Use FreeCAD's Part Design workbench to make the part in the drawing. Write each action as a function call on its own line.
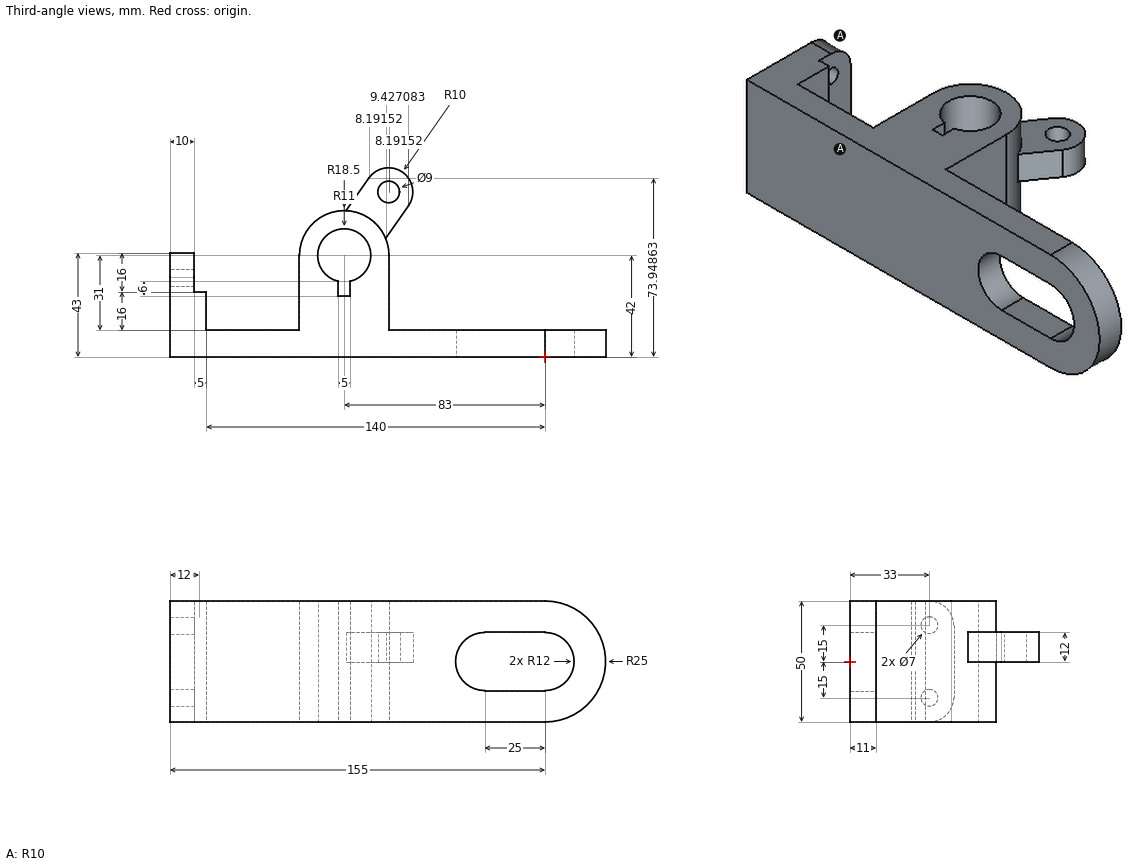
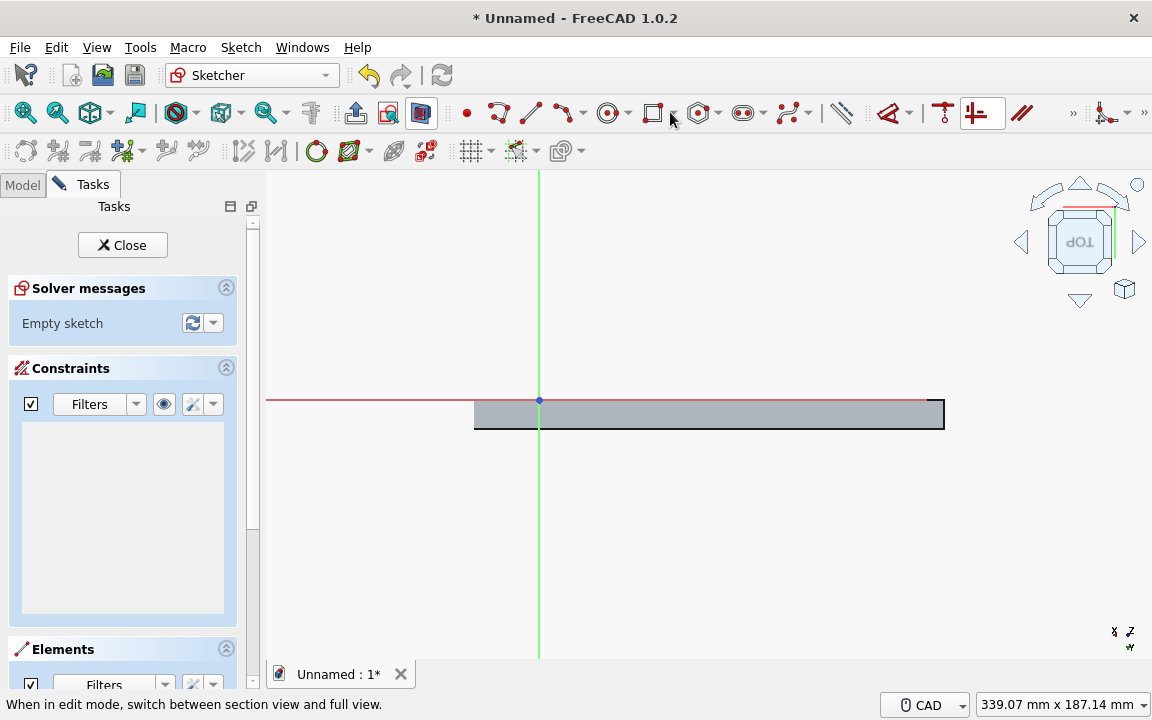
click(500, 114)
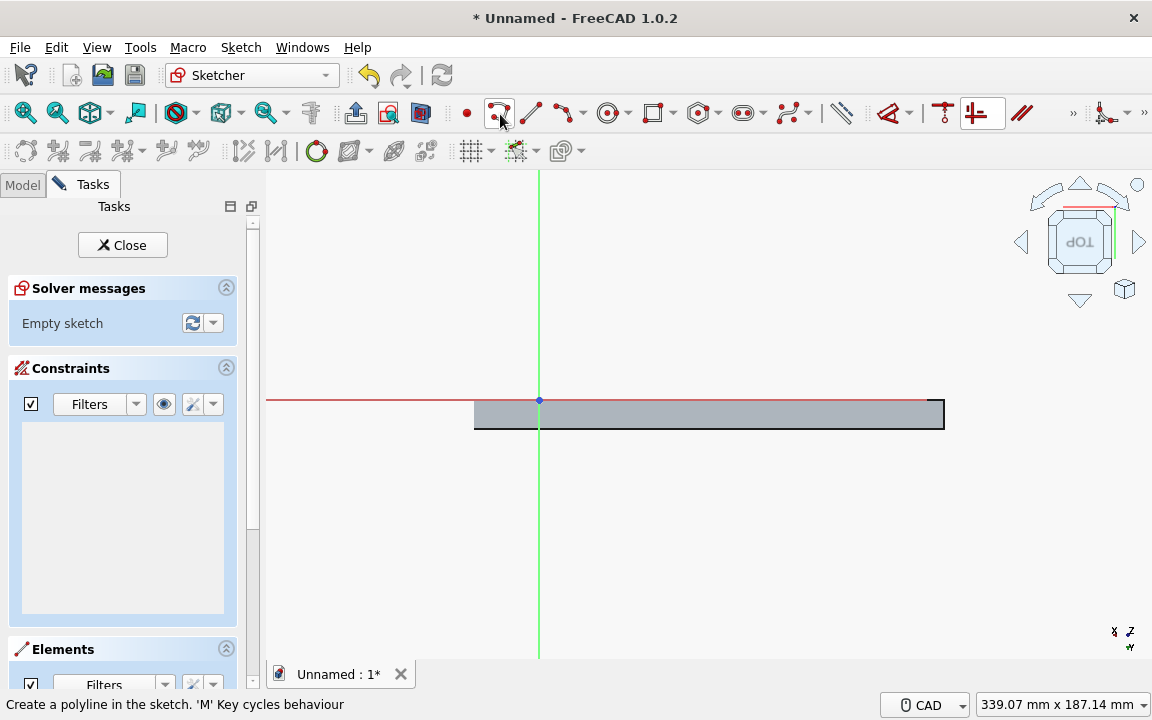
click(905, 429)
click(905, 471)
click(918, 471)
click(918, 512)
click(944, 512)
click(944, 400)
click(905, 430)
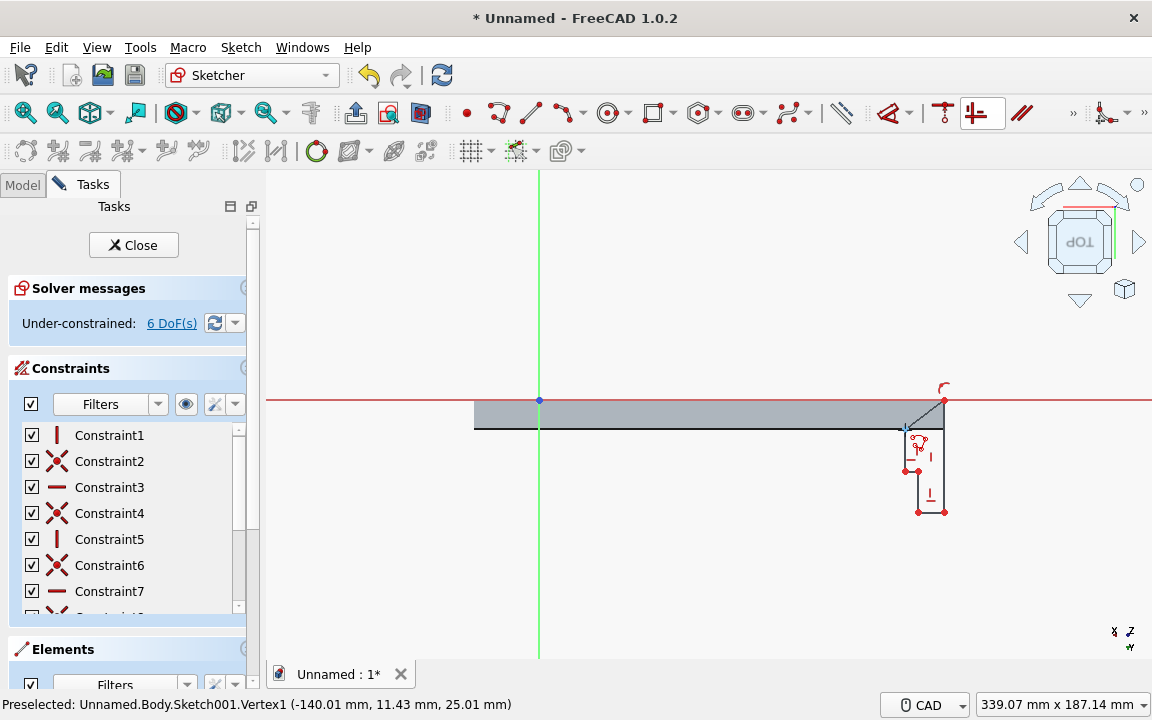
click(804, 510)
click(804, 429)
click(708, 429)
click(708, 510)
right_click(708, 510)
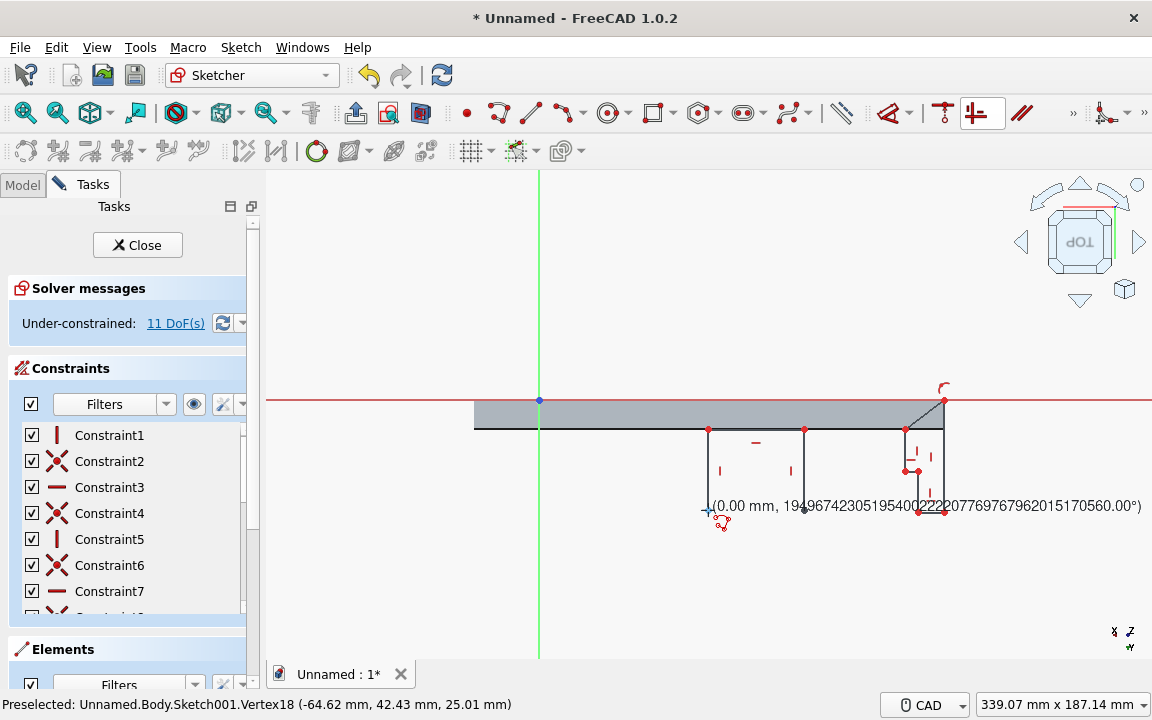
click(564, 114)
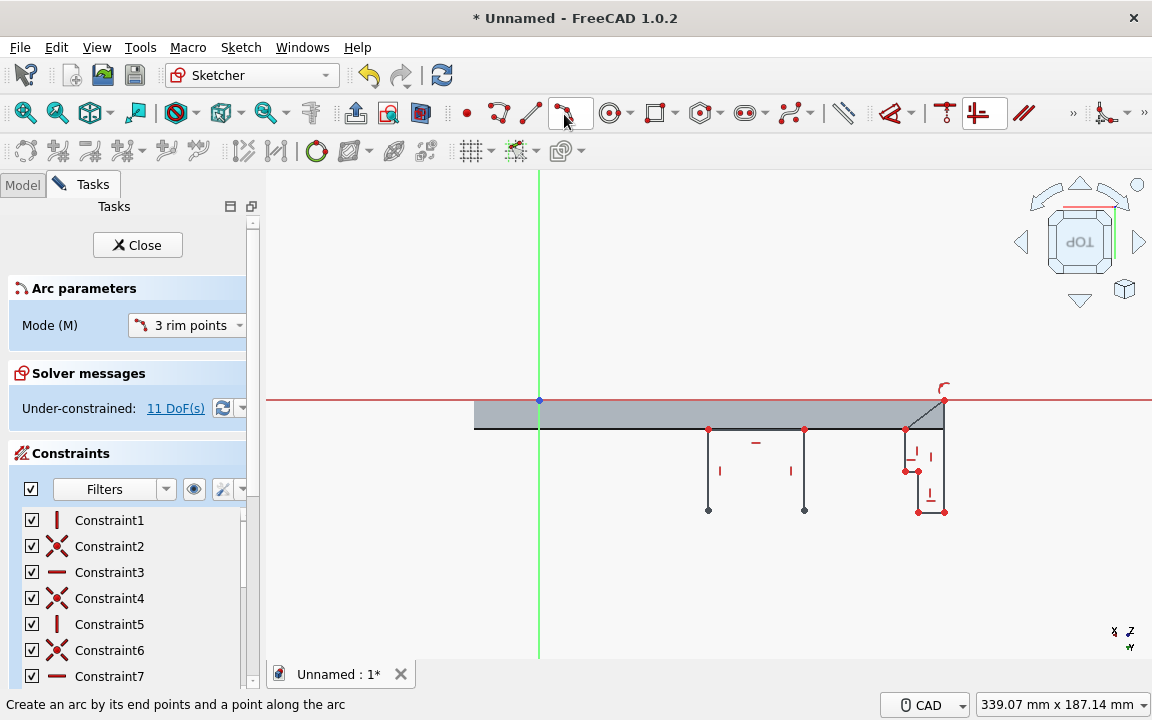
click(708, 511)
click(804, 511)
click(756, 558)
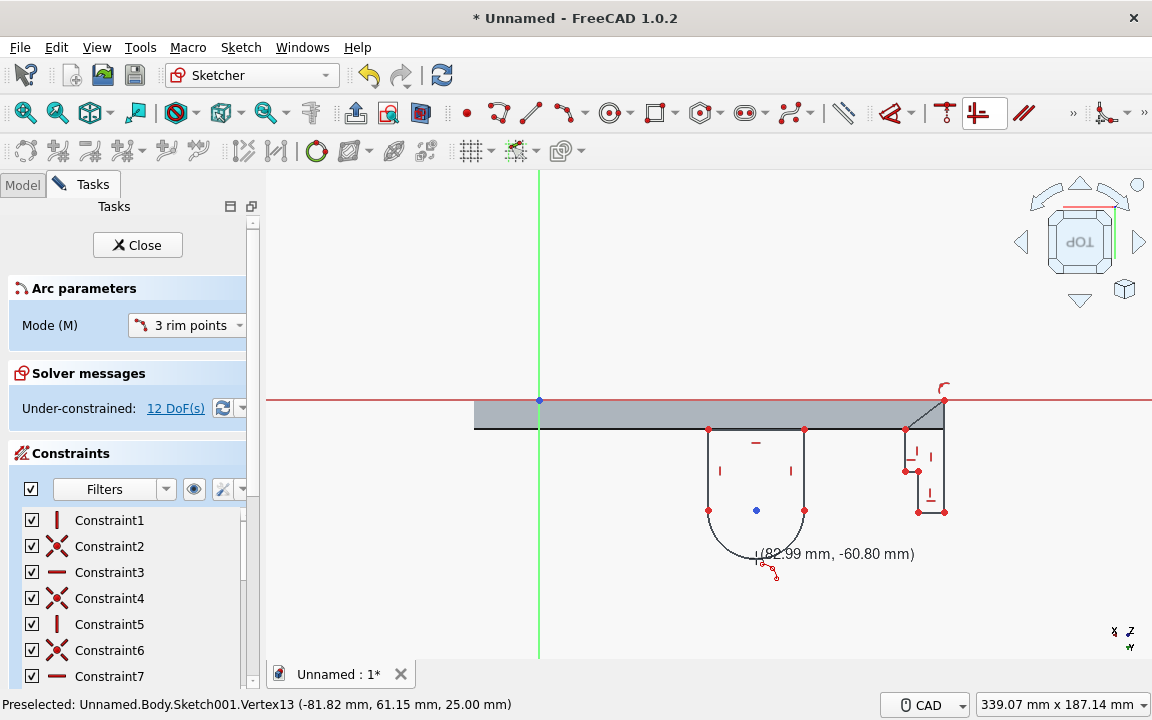
click(500, 114)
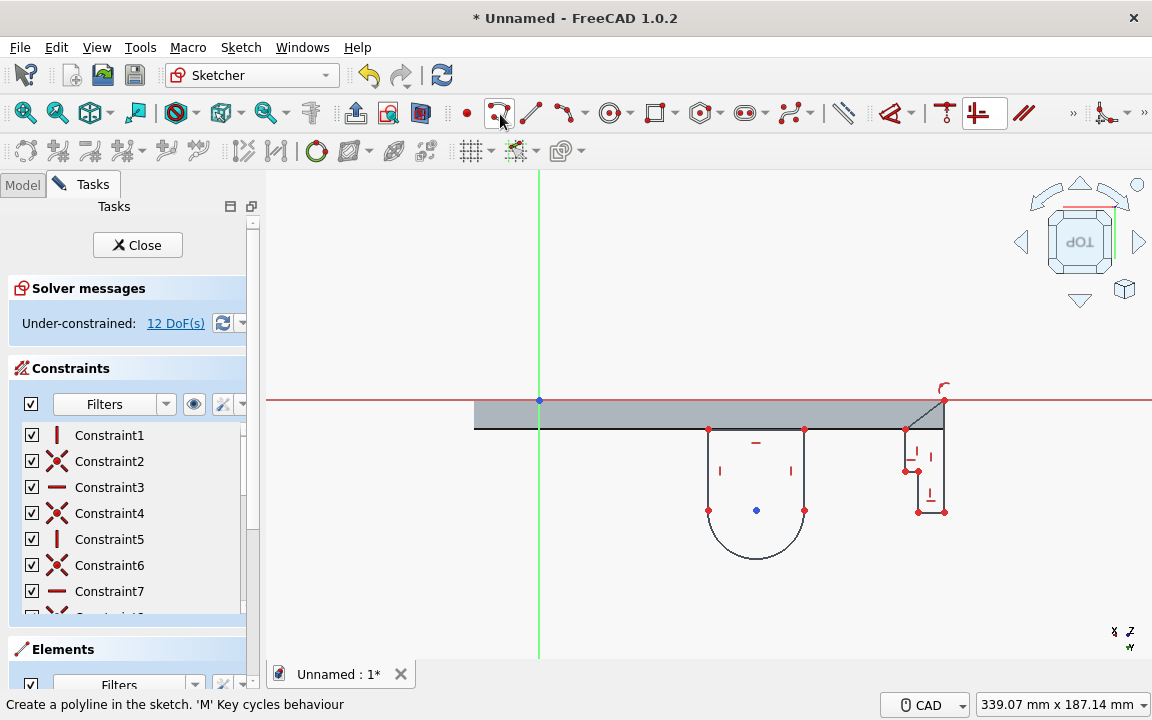
click(750, 482)
click(750, 466)
click(763, 466)
click(763, 482)
right_click(763, 482)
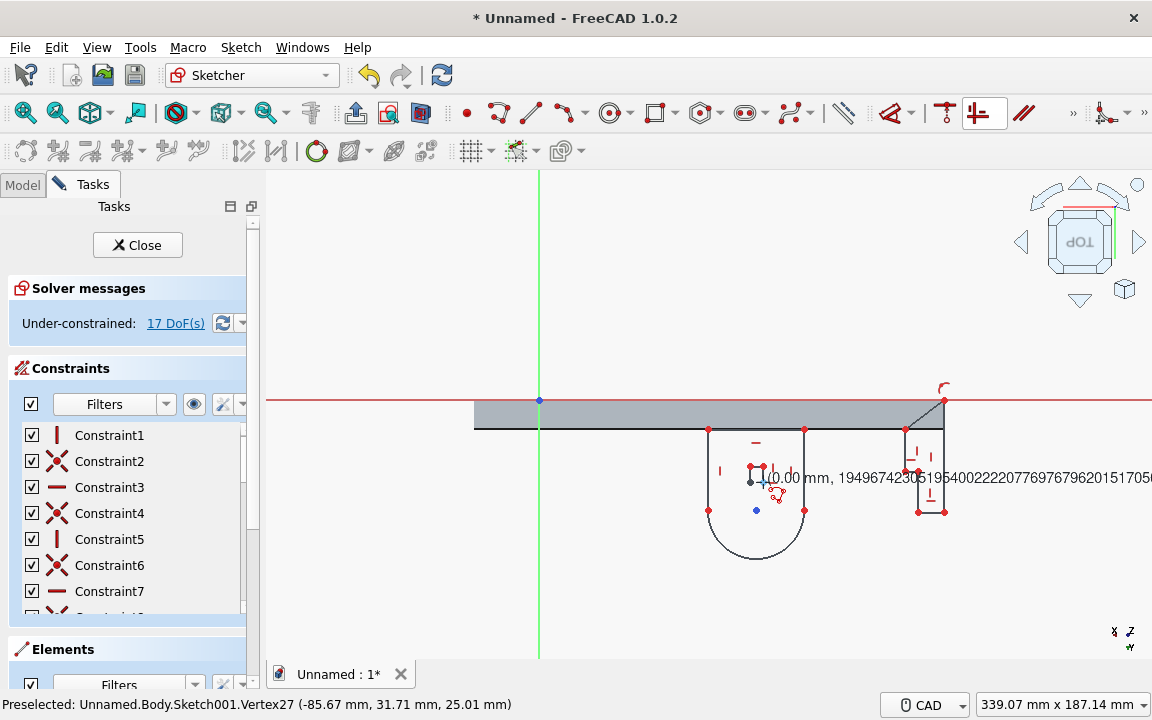
key(g)
key(3)
key(a)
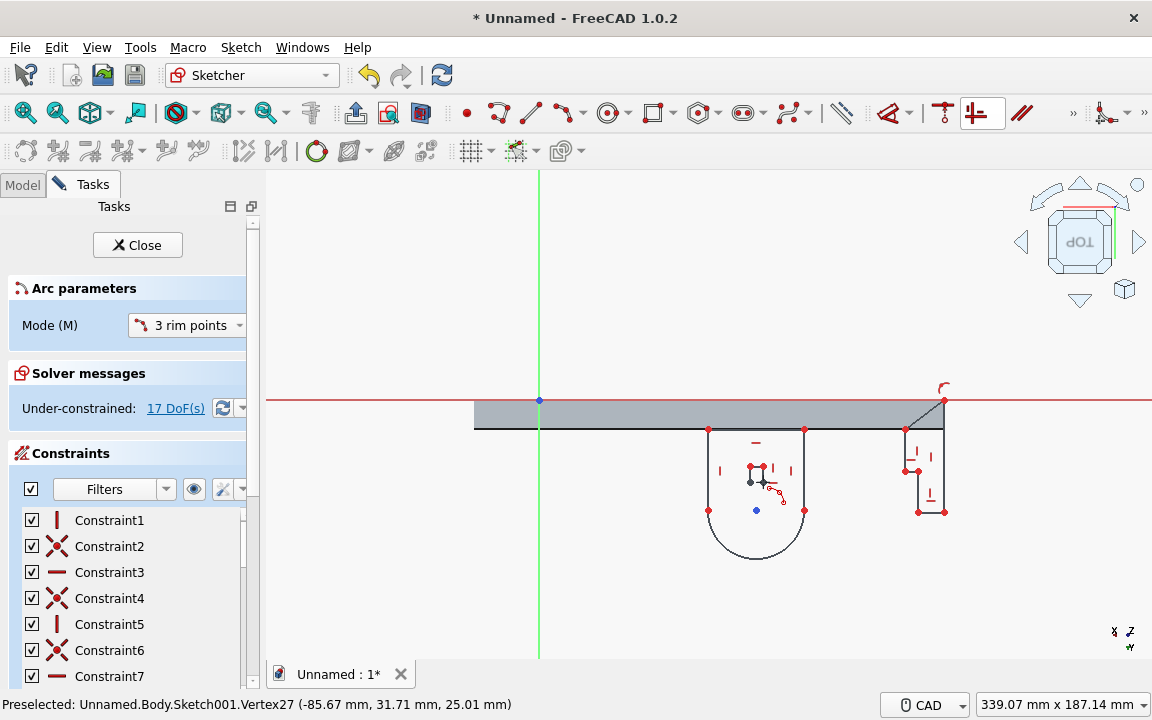
scroll(763, 482, up, 4)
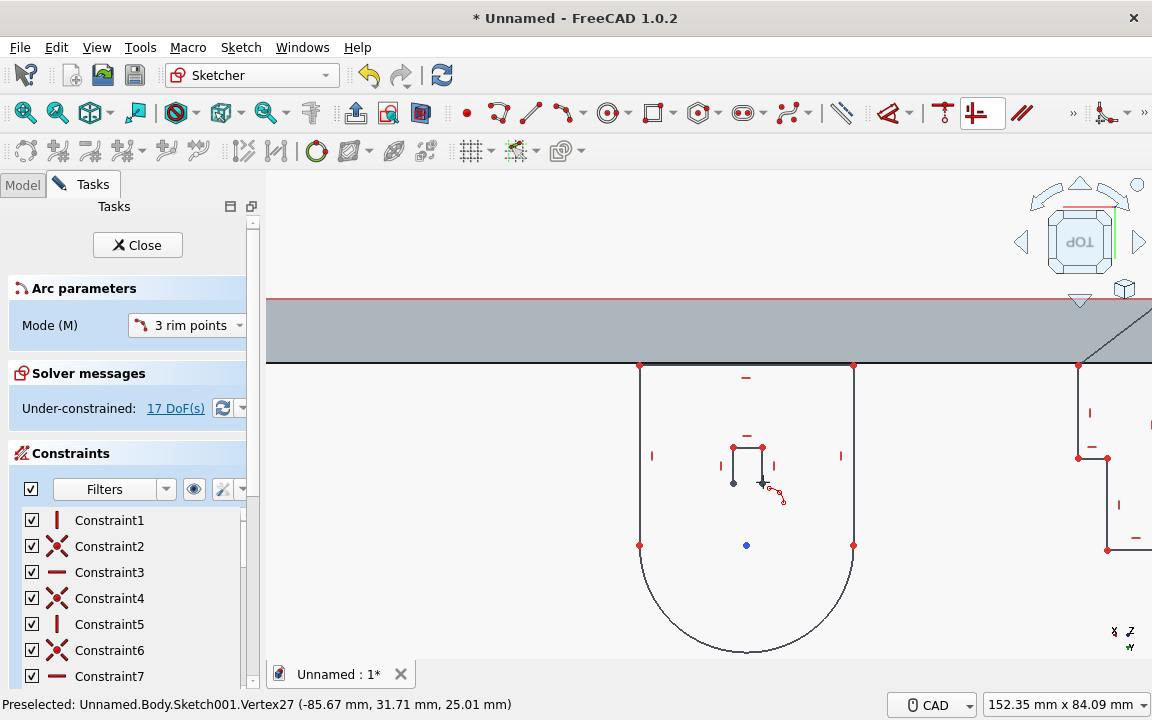
click(762, 483)
click(733, 483)
click(747, 607)
key(Escape)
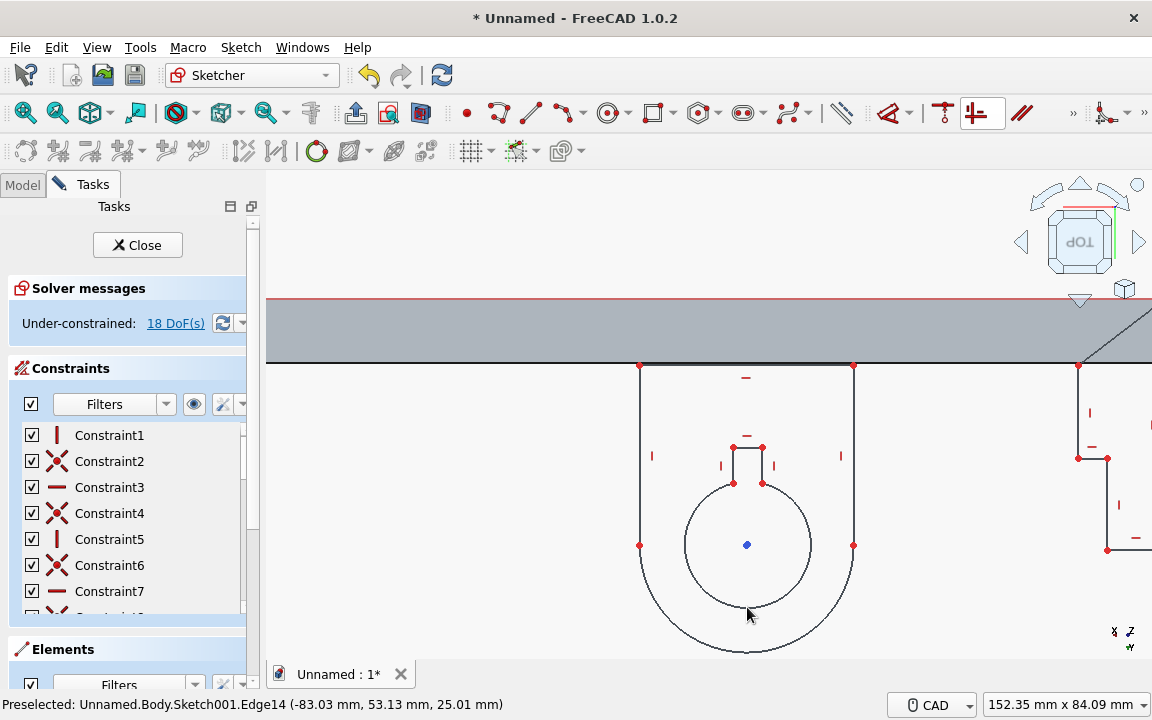
click(854, 492)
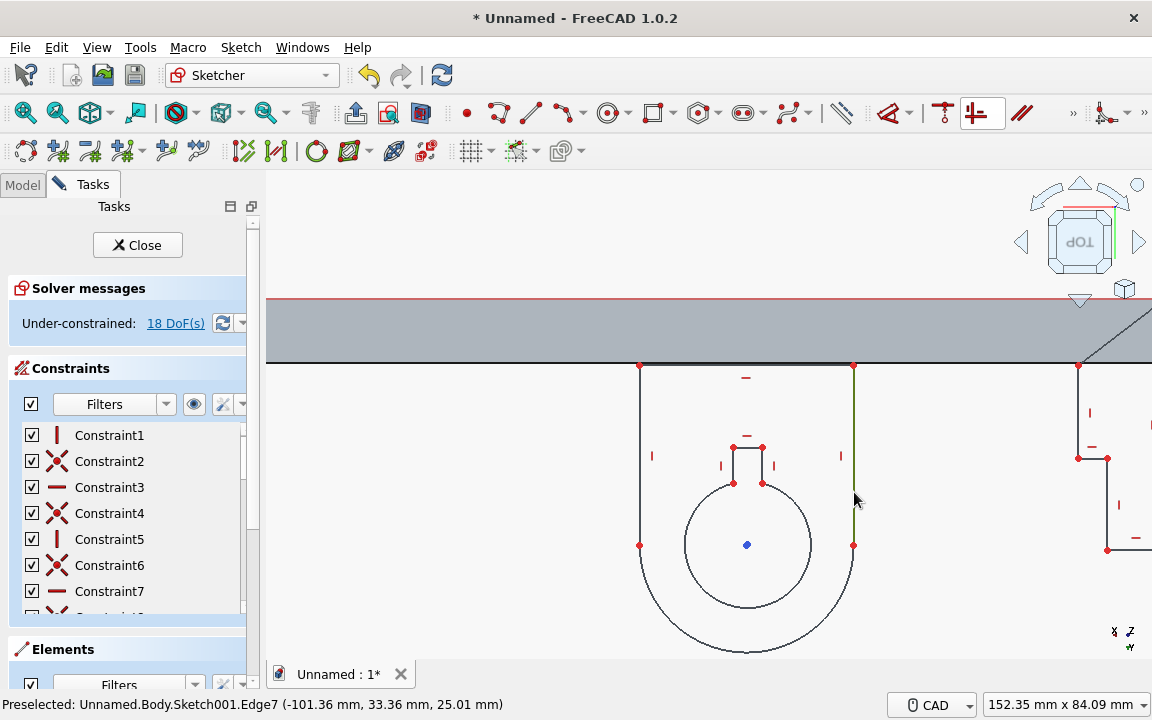
click(660, 609)